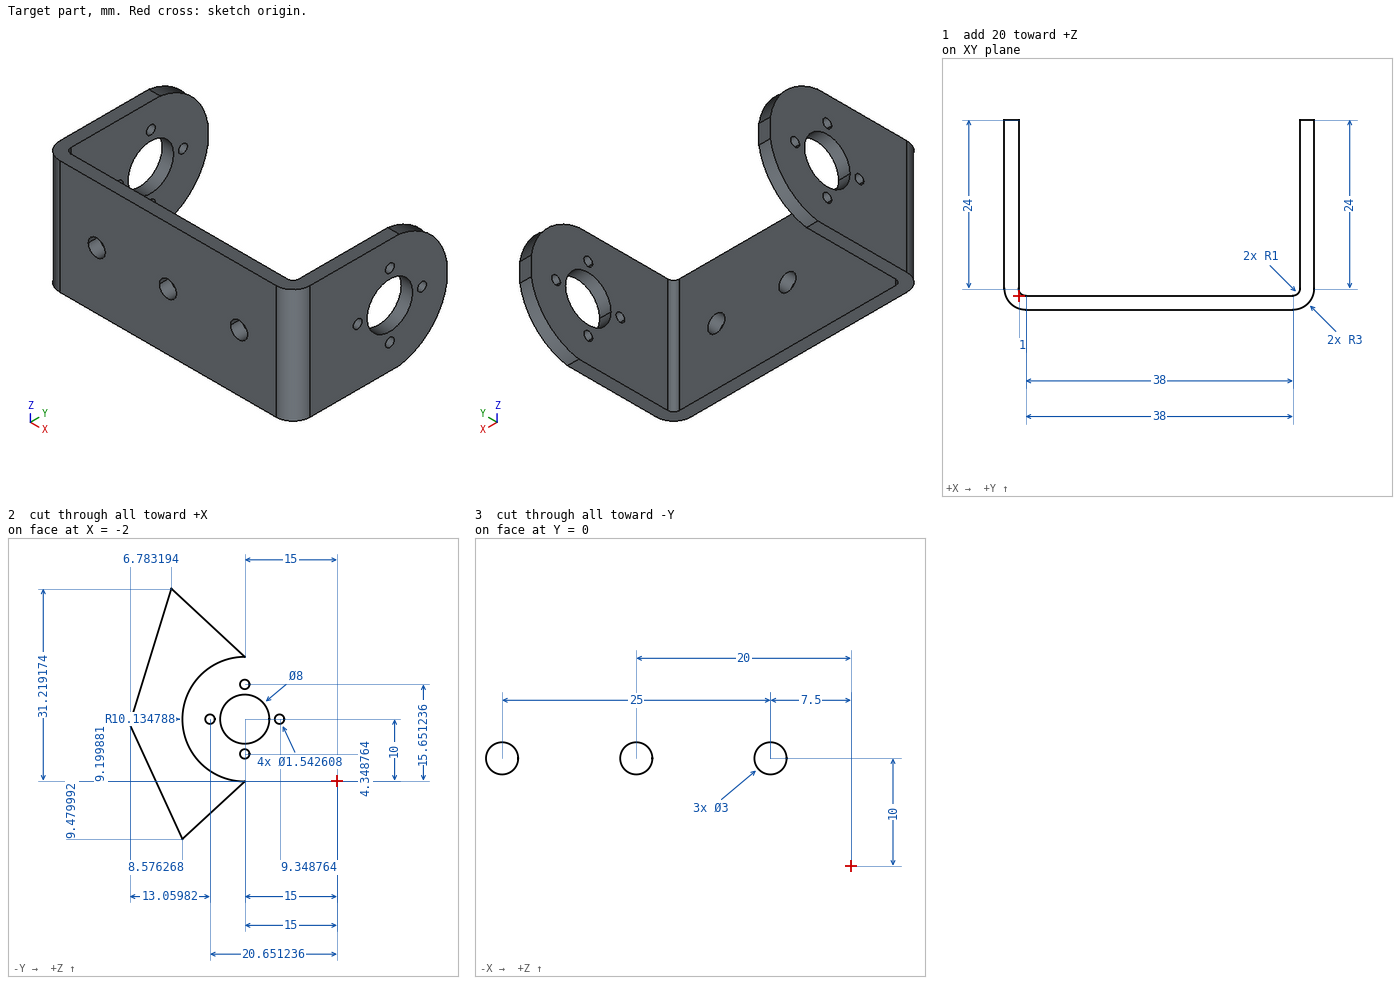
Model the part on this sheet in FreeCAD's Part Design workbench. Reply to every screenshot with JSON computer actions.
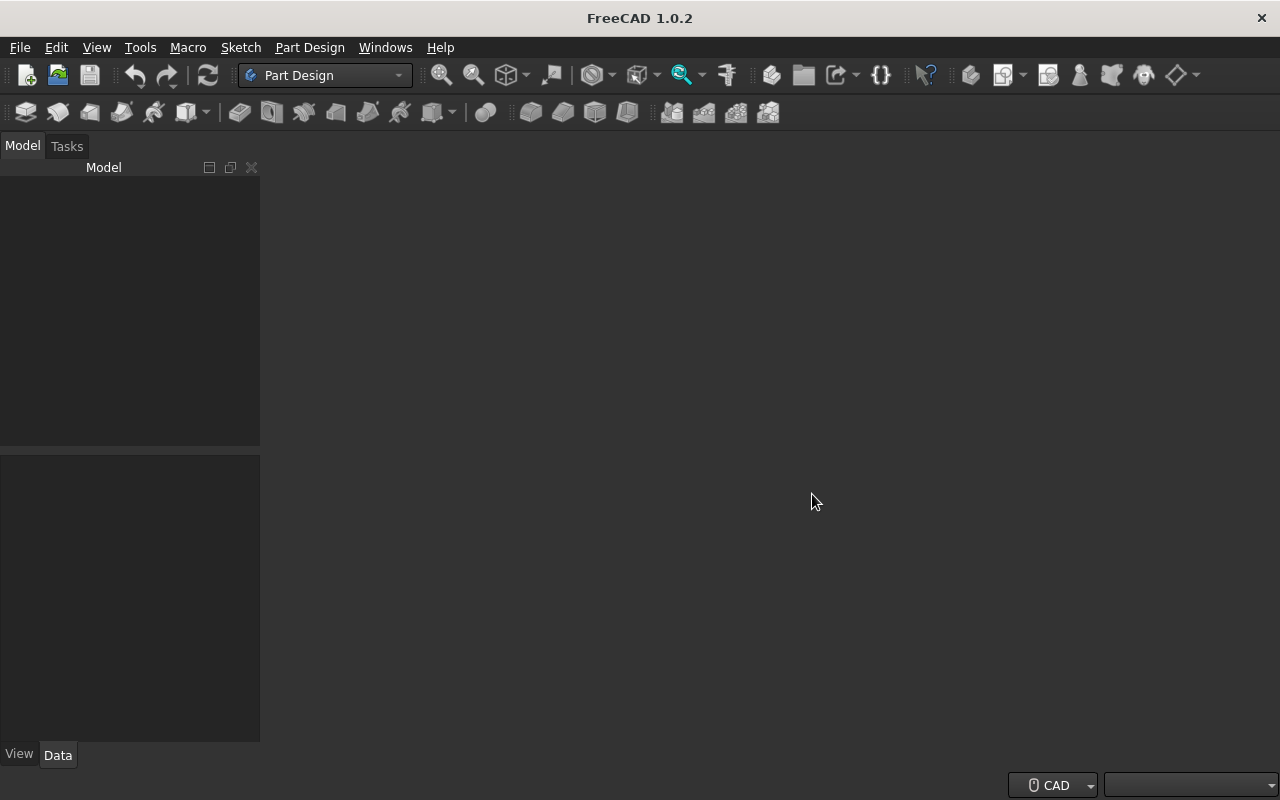
{"action": "left_click", "coordinate": [26, 76]}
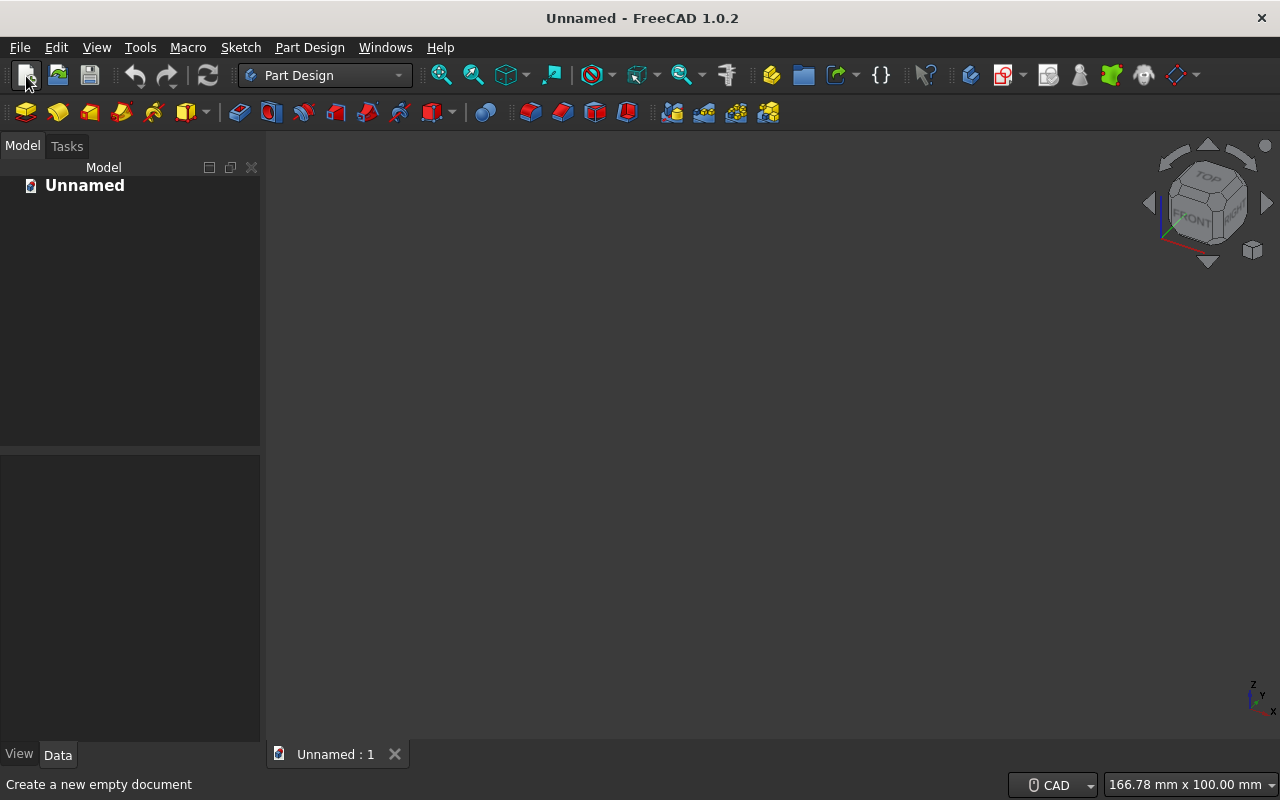
{"action": "left_click", "coordinate": [1004, 76]}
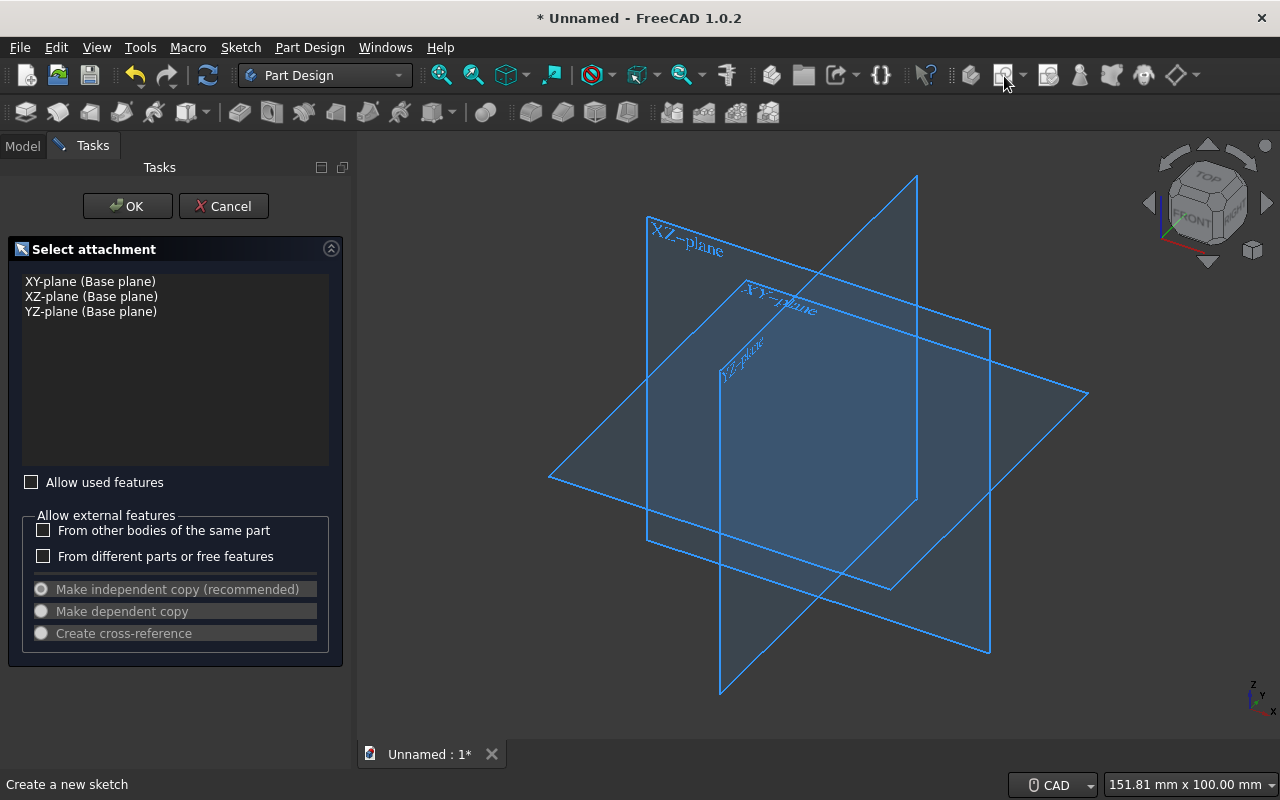
{"action": "left_click", "coordinate": [82, 282]}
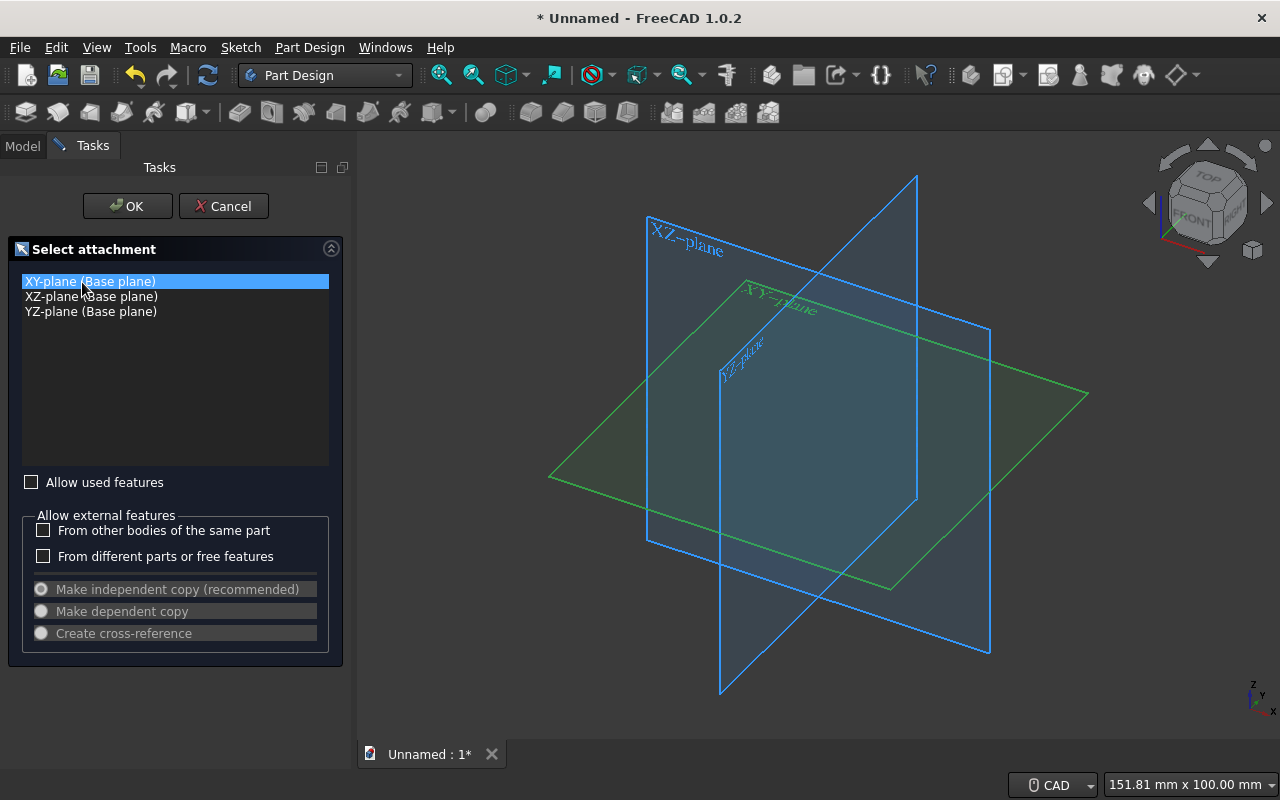
{"action": "left_click", "coordinate": [128, 206]}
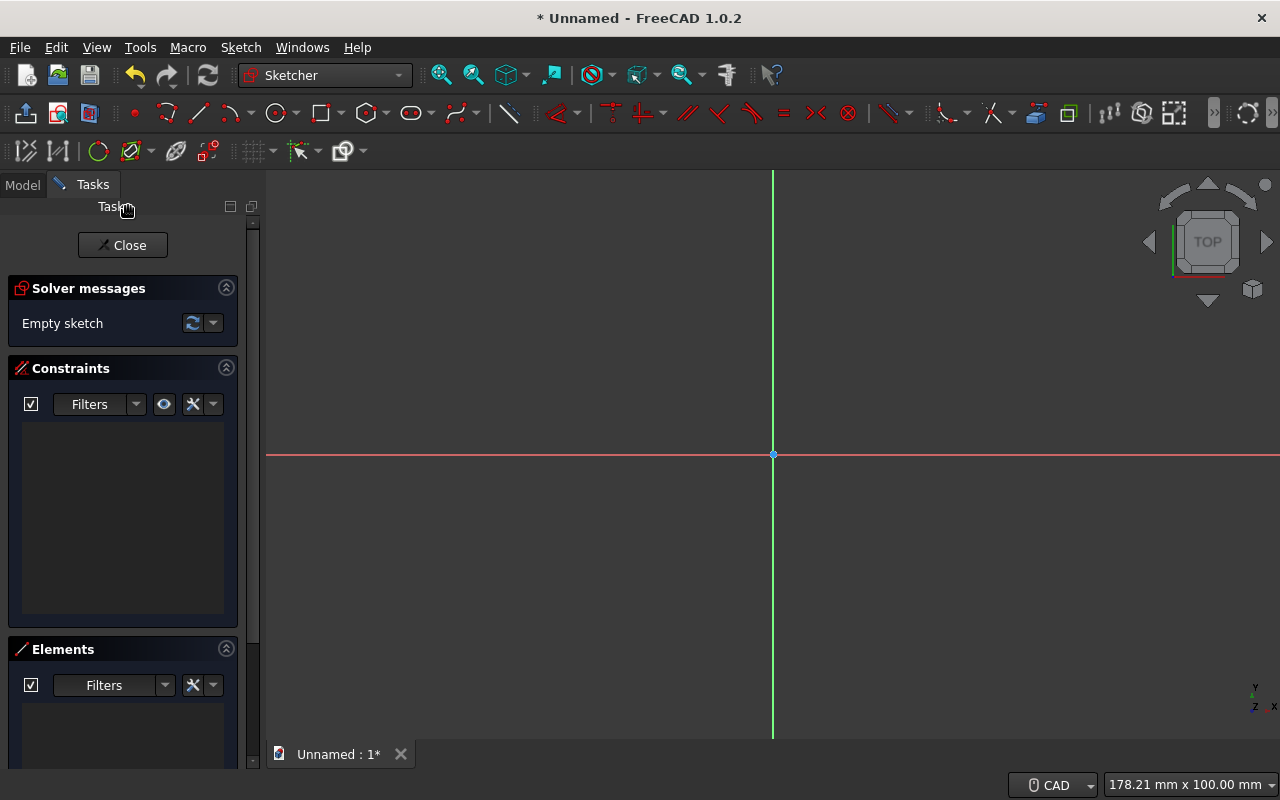
{"action": "scroll", "coordinate": [1036, 336], "scroll_direction": "up", "scroll_amount": 4}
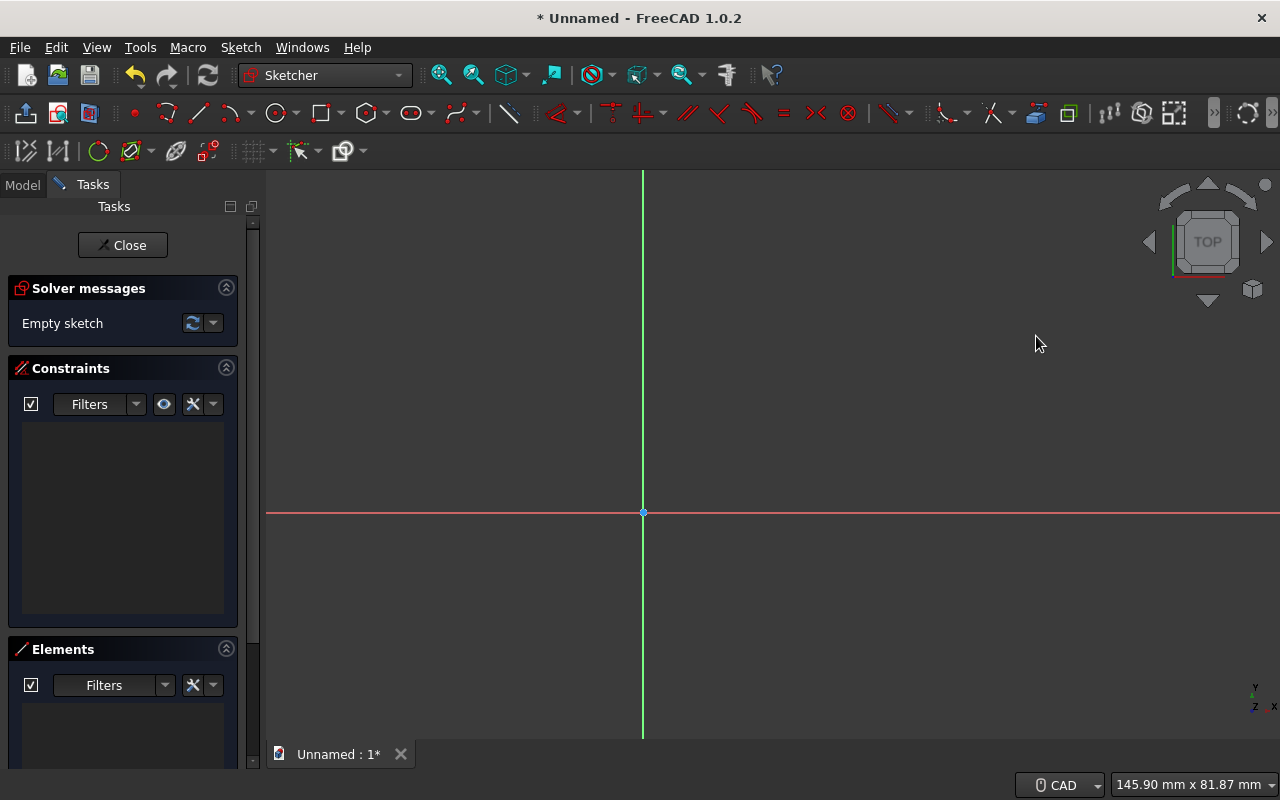
{"action": "left_click", "coordinate": [168, 114]}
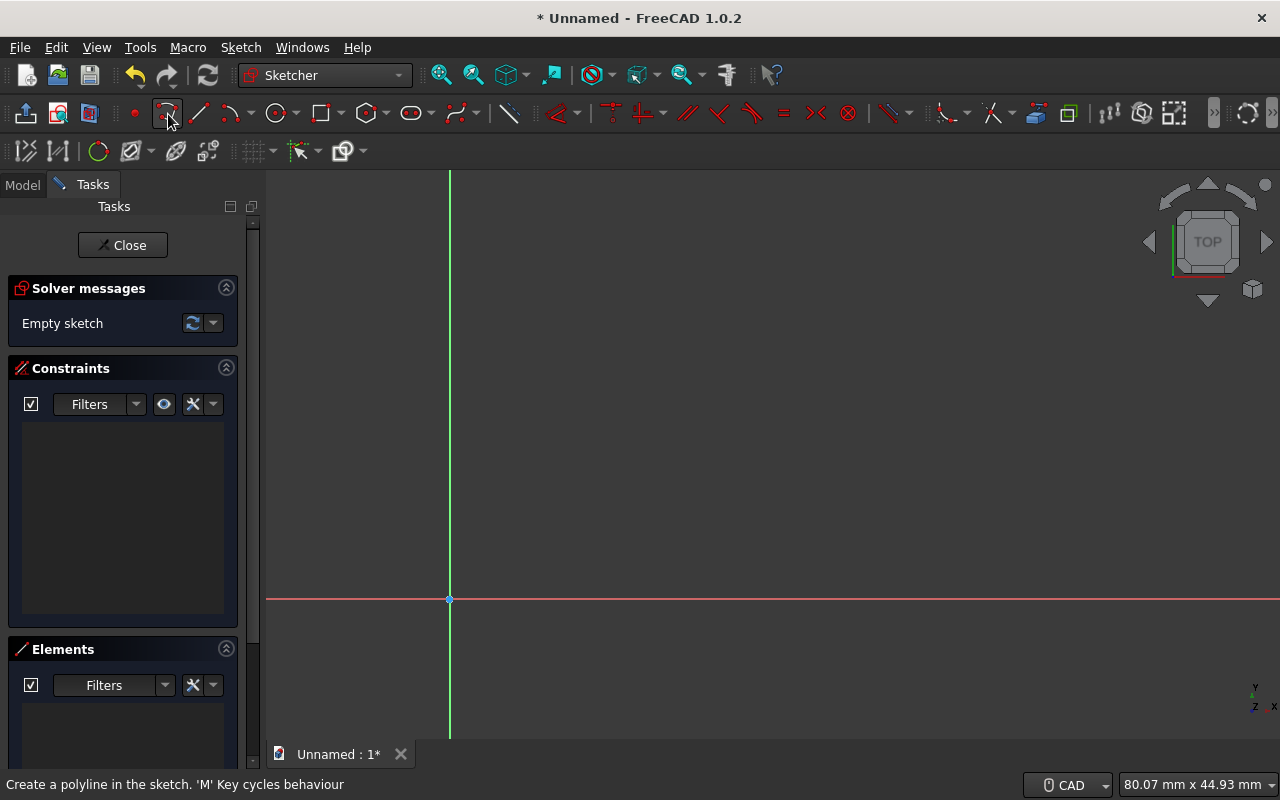
{"action": "scroll", "coordinate": [450, 587], "scroll_direction": "up", "scroll_amount": 2}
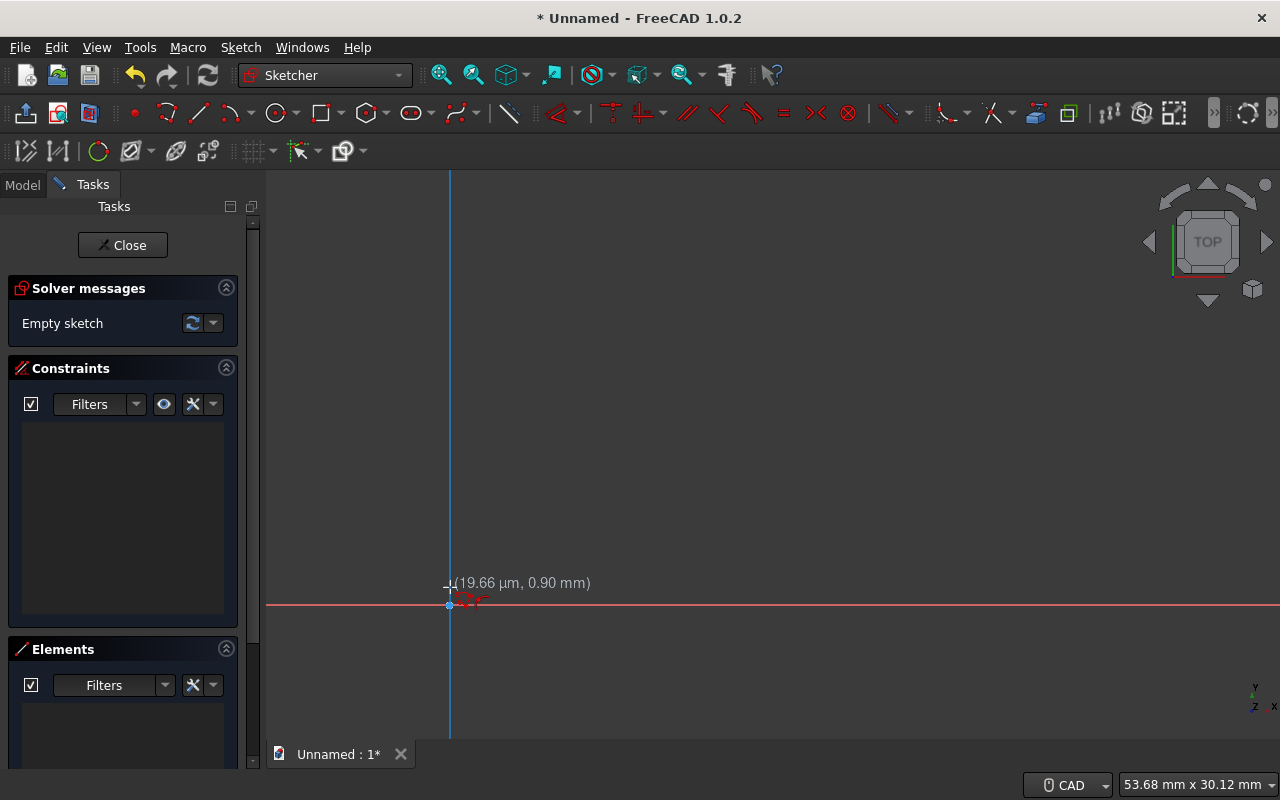
{"action": "left_click", "coordinate": [450, 586]}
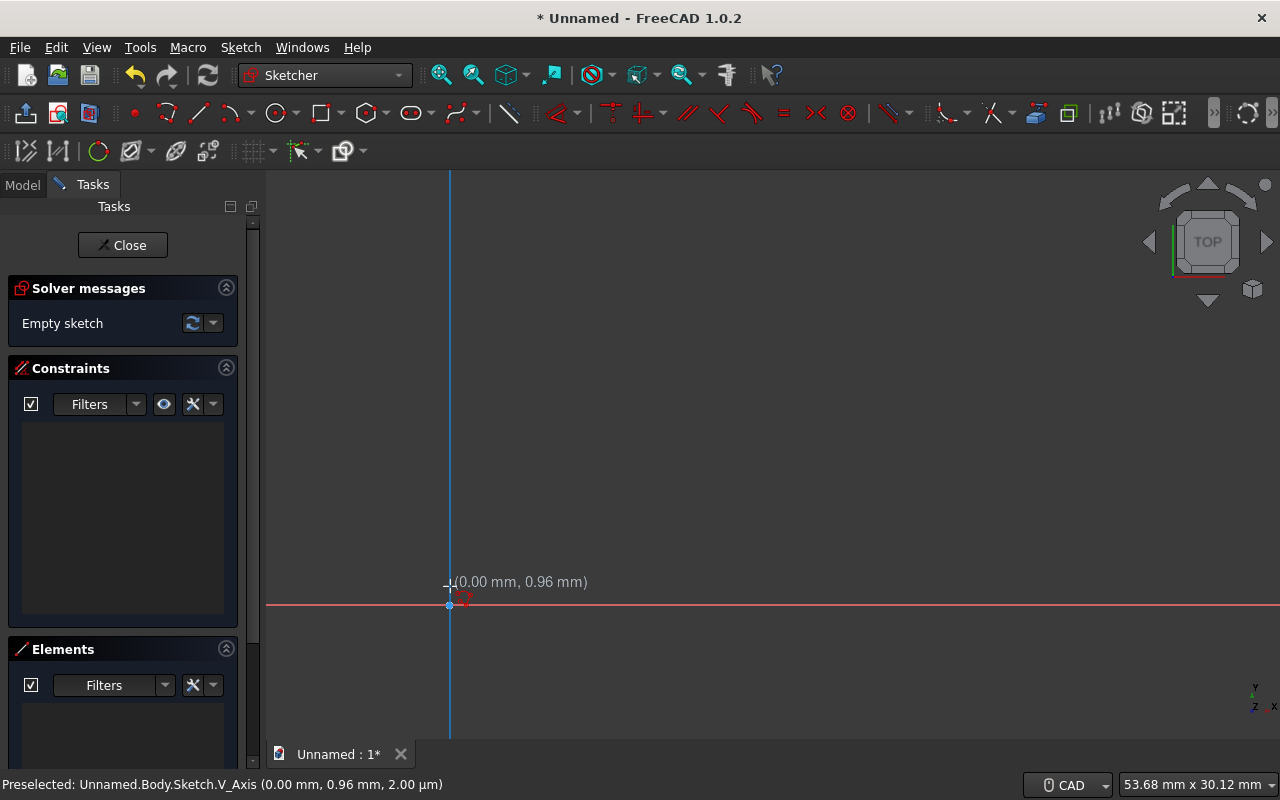
{"action": "scroll", "coordinate": [455, 590], "scroll_direction": "down", "scroll_amount": 2}